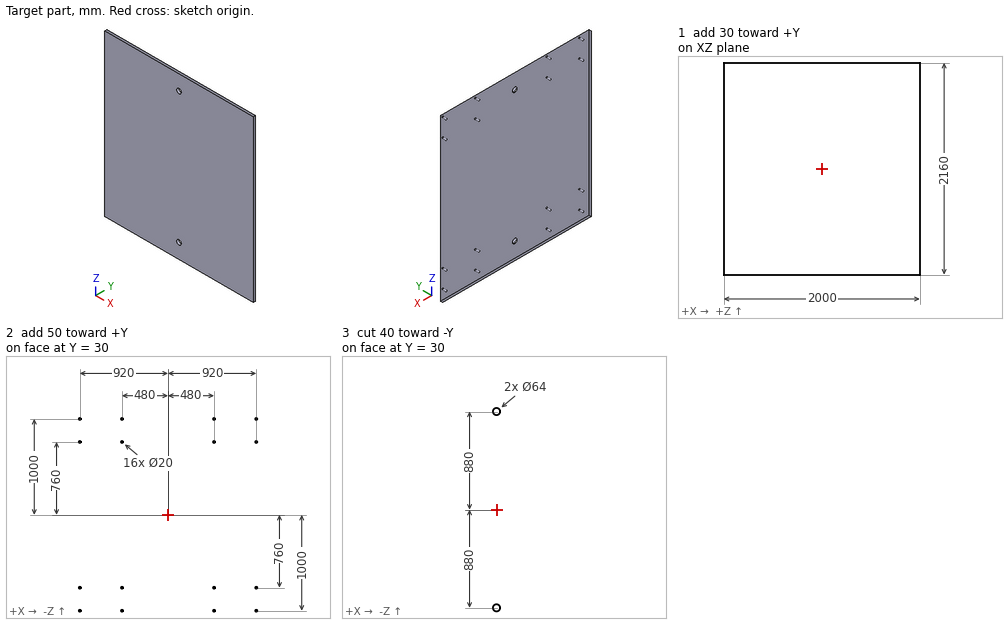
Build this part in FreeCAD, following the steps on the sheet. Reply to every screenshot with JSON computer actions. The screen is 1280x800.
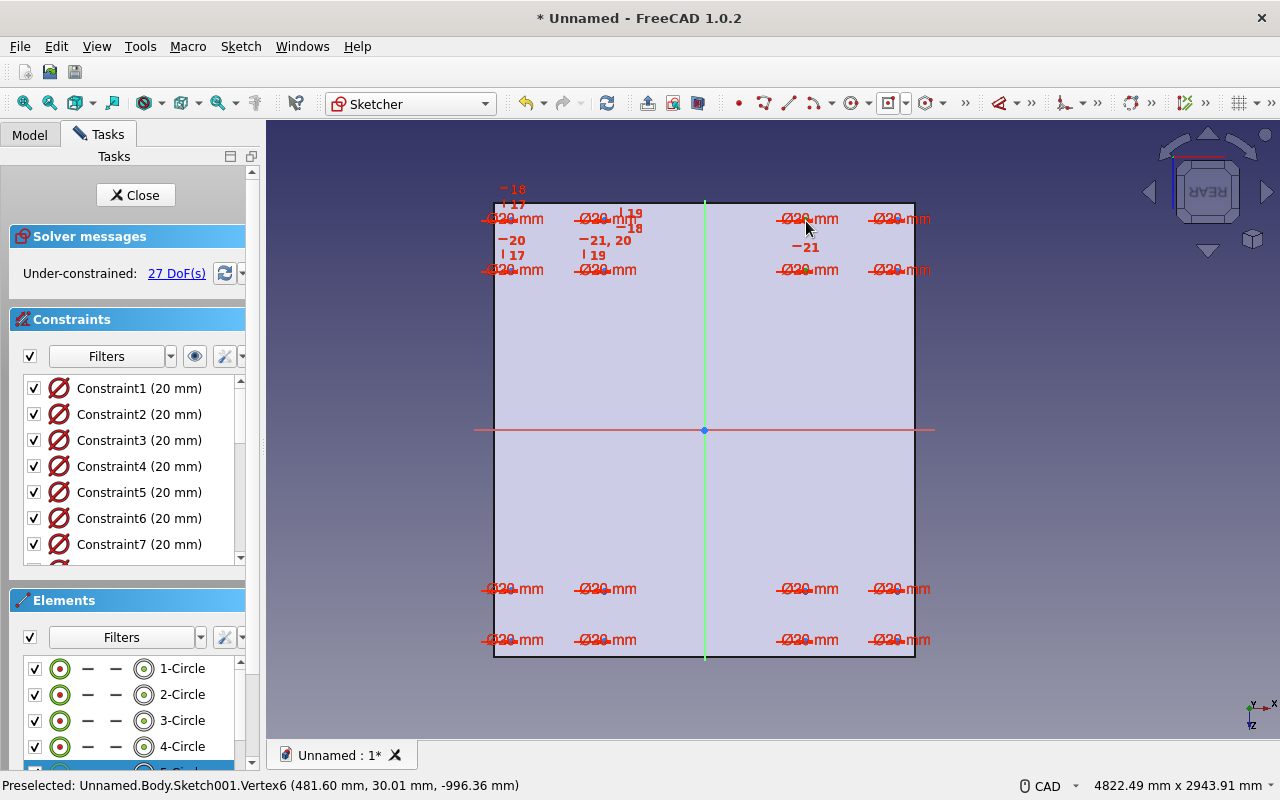
{"action": "key", "text": "v"}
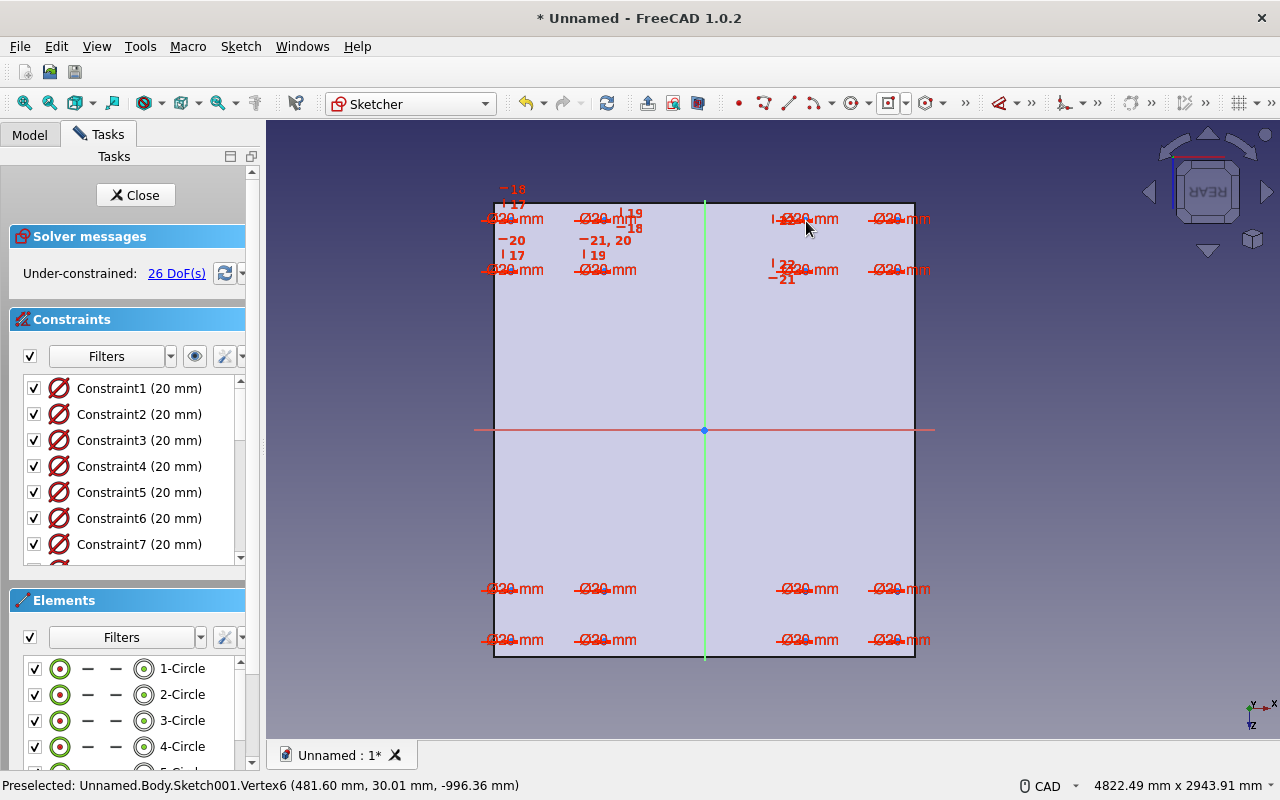
{"action": "left_click", "coordinate": [604, 221]}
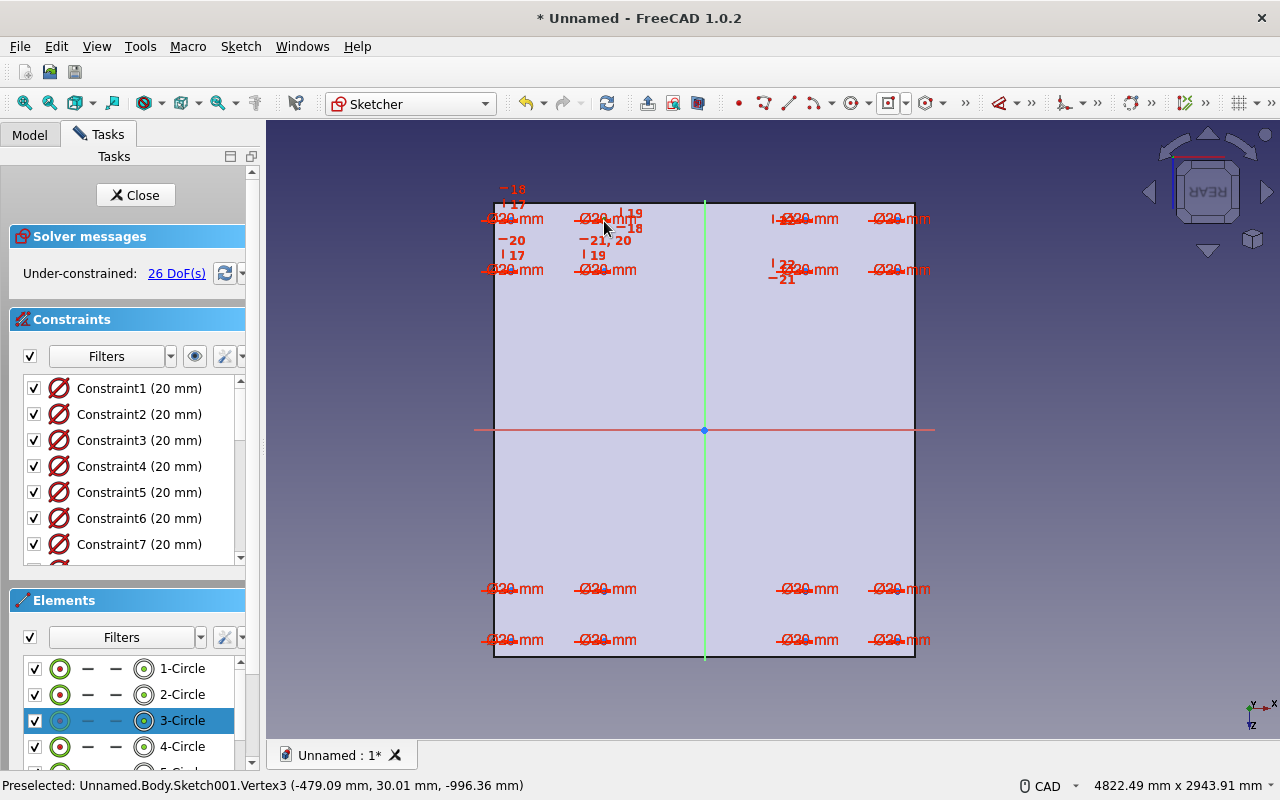
{"action": "left_click", "coordinate": [806, 221]}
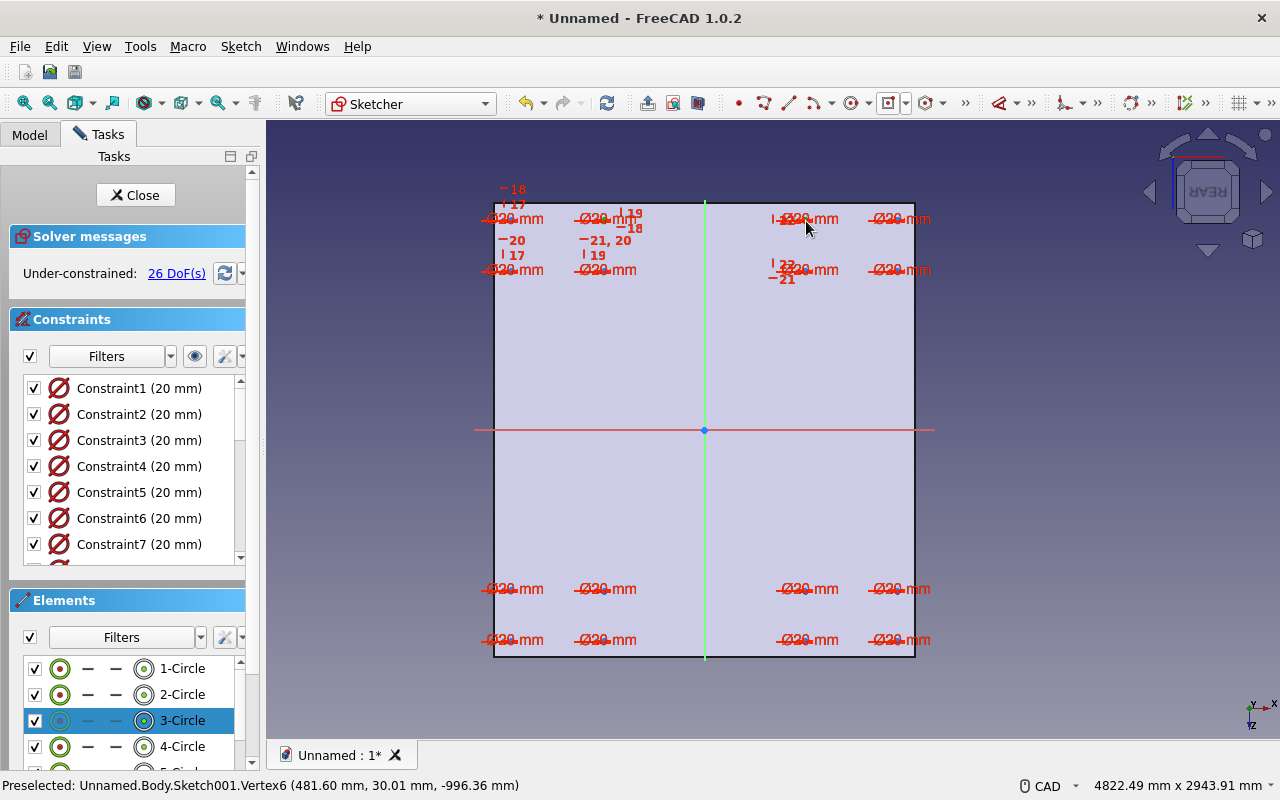
{"action": "key", "text": "h"}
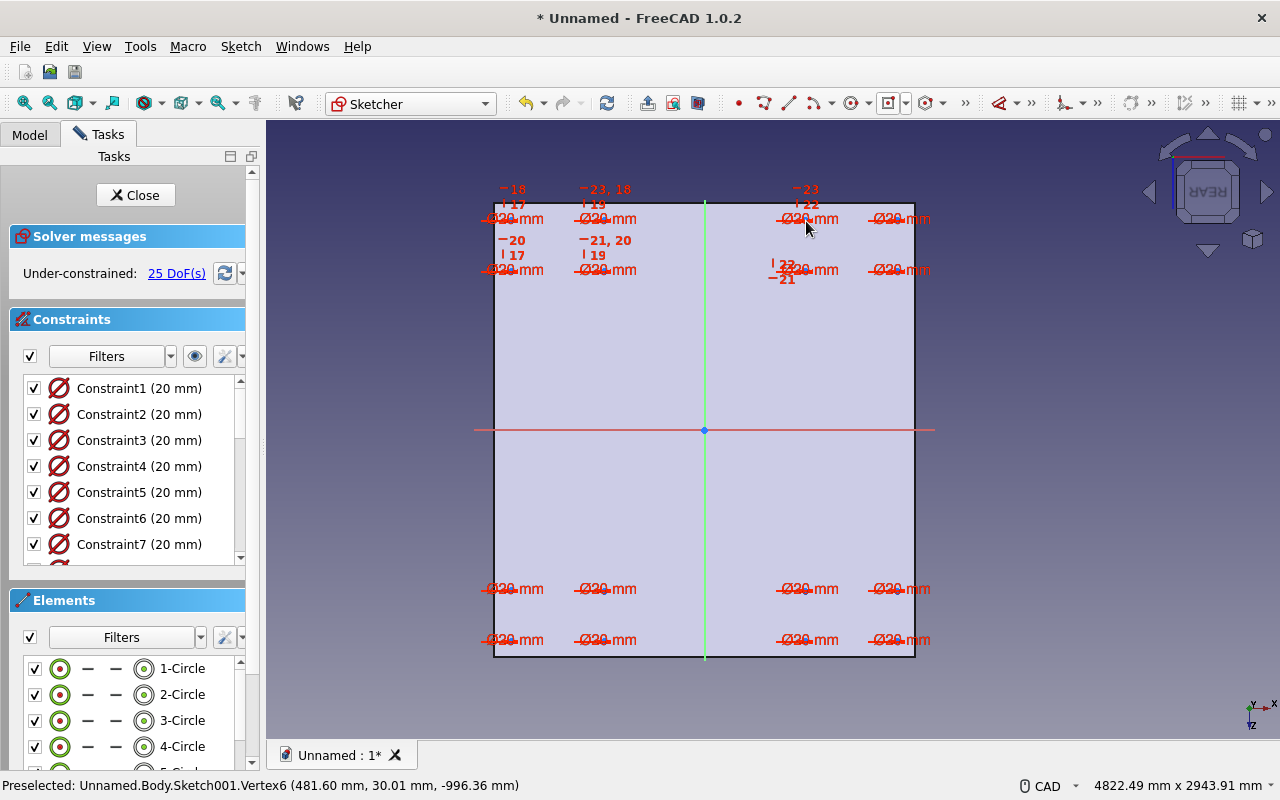
{"action": "left_click", "coordinate": [806, 272]}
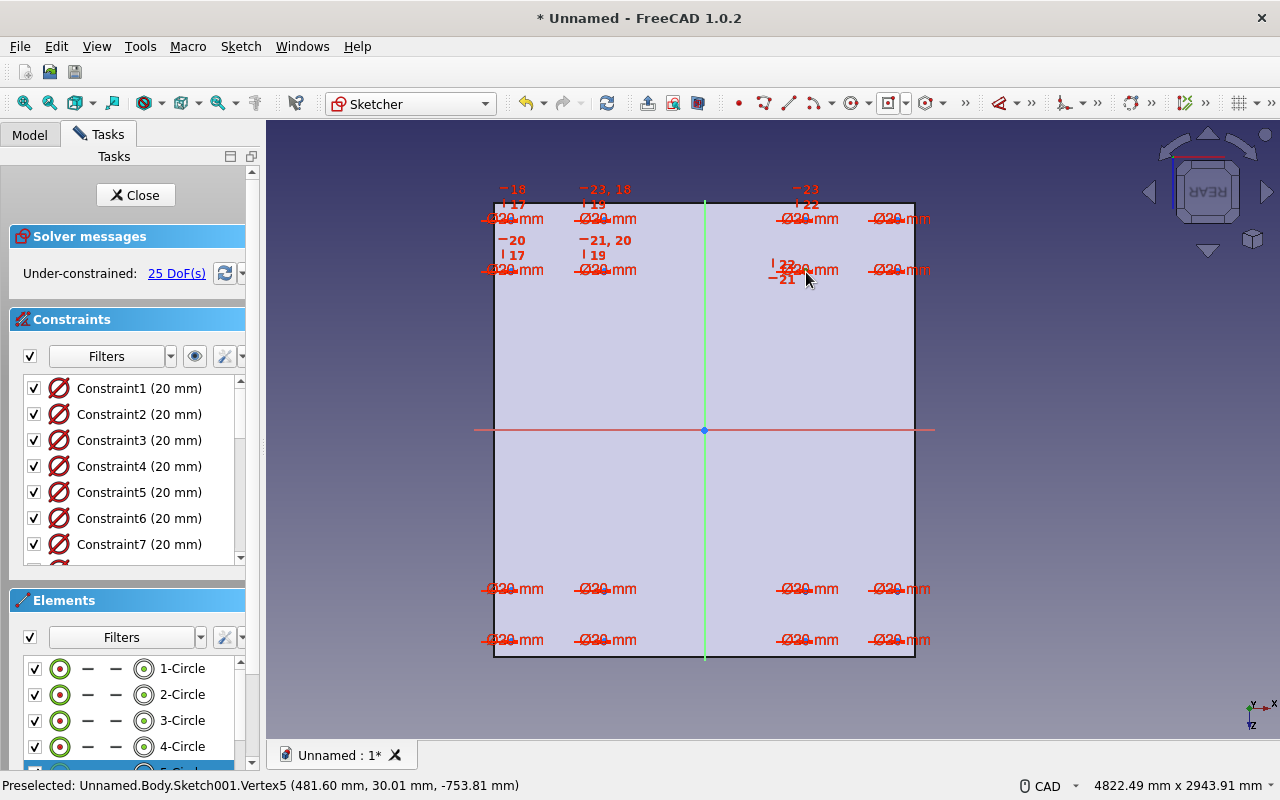
{"action": "left_click", "coordinate": [898, 272]}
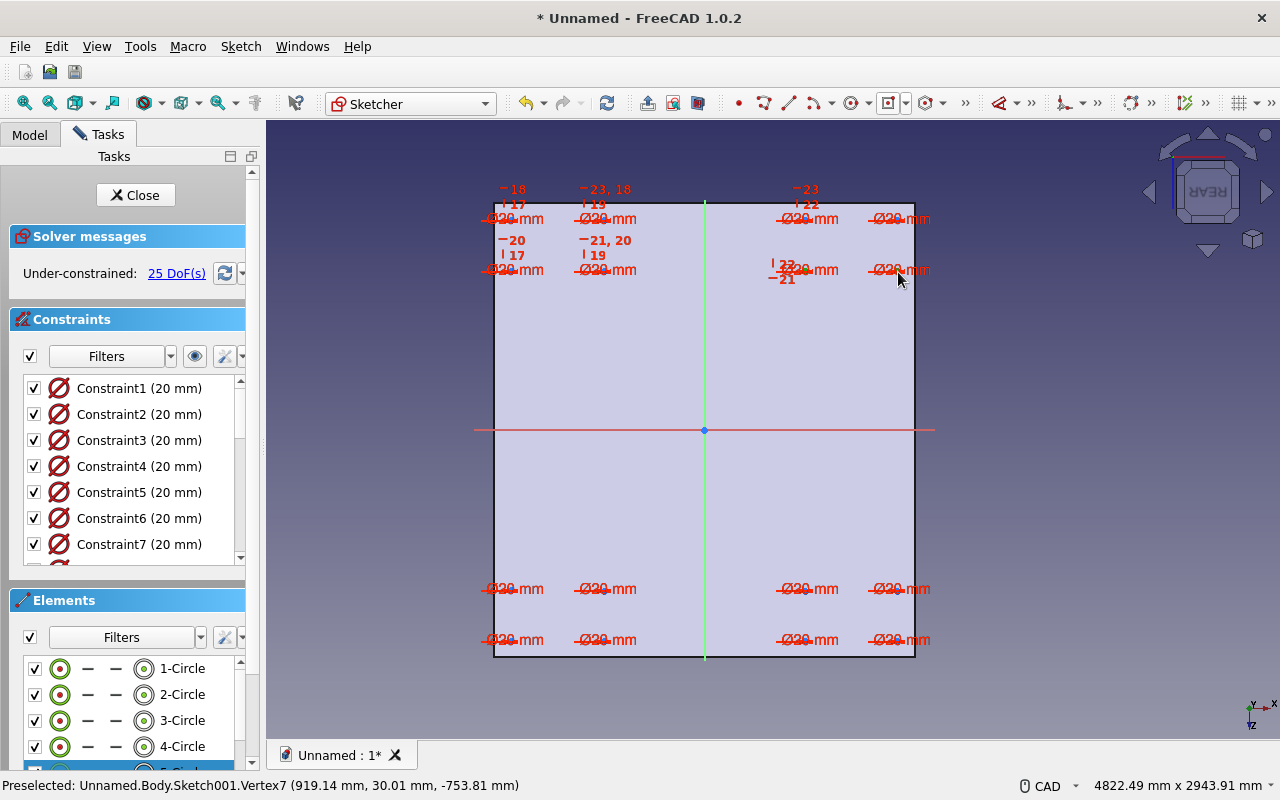
{"action": "key", "text": "h"}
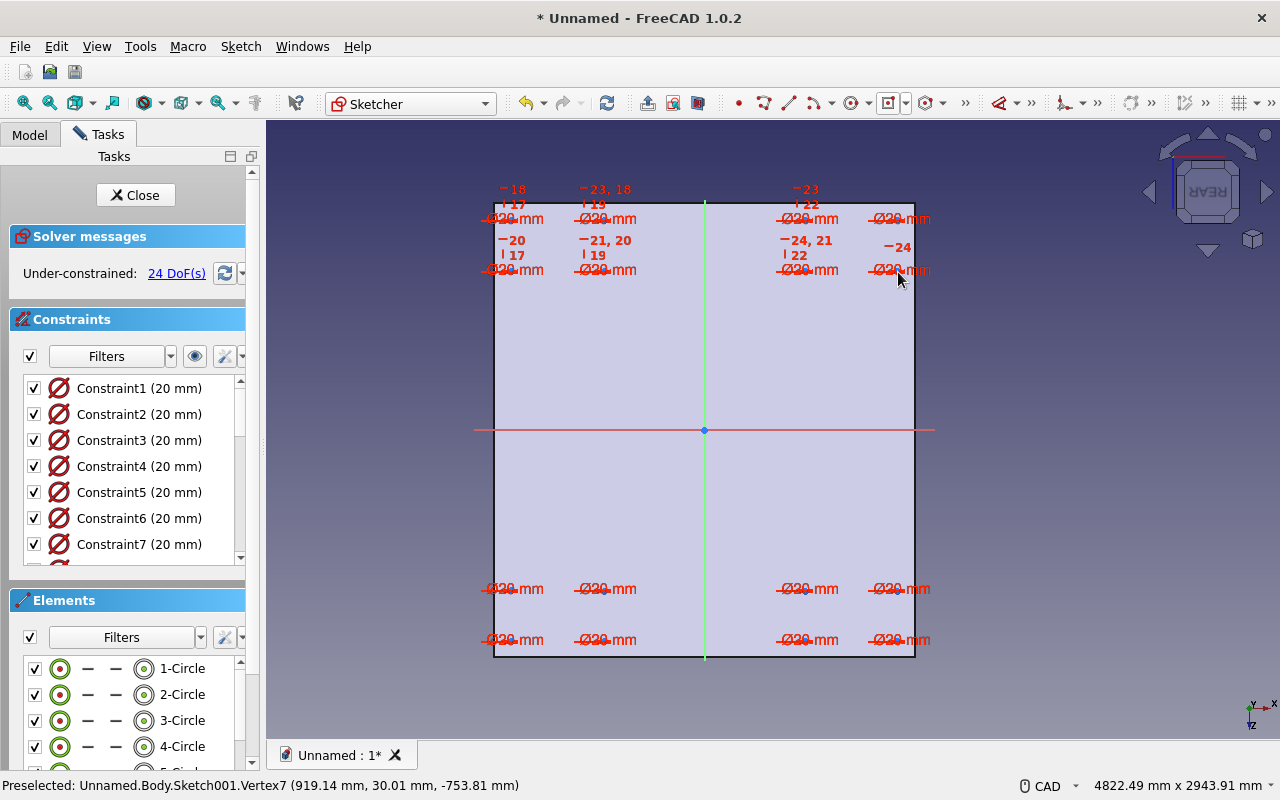
{"action": "left_click", "coordinate": [898, 272]}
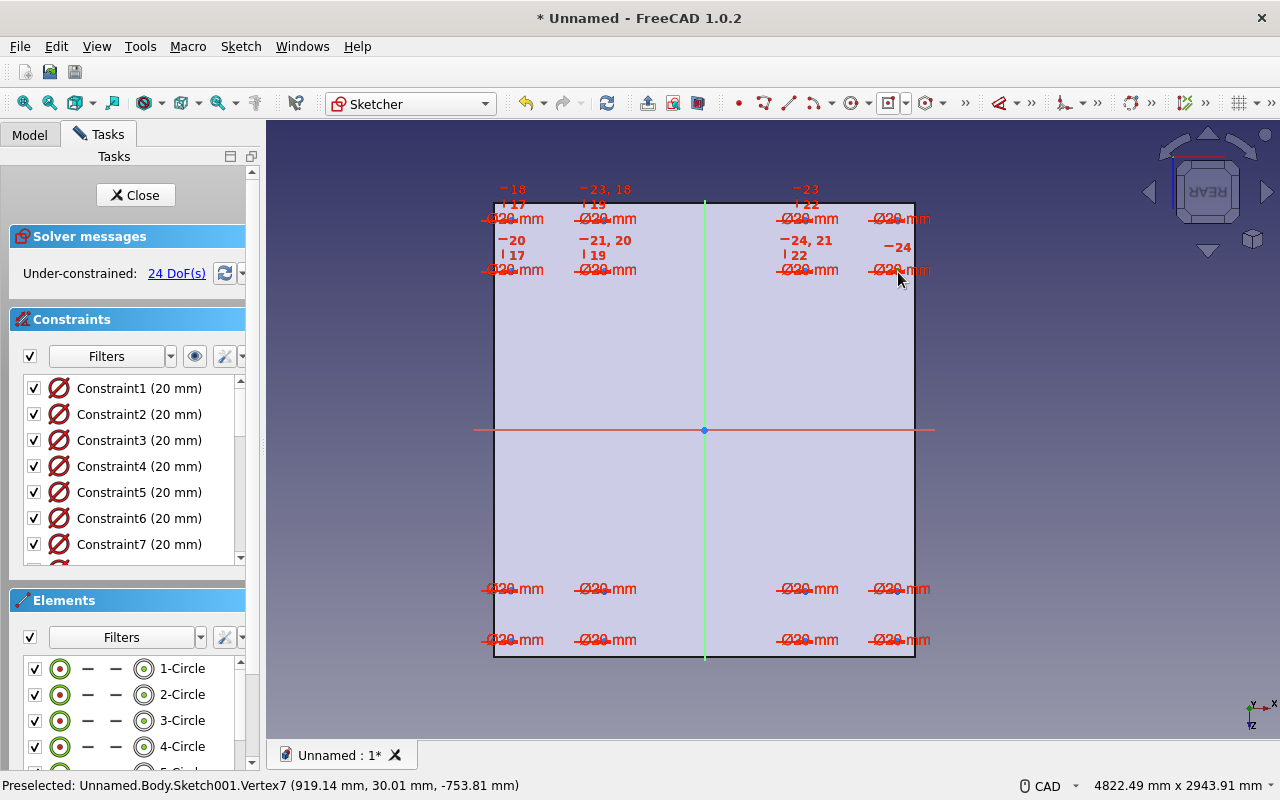
{"action": "left_click", "coordinate": [898, 221]}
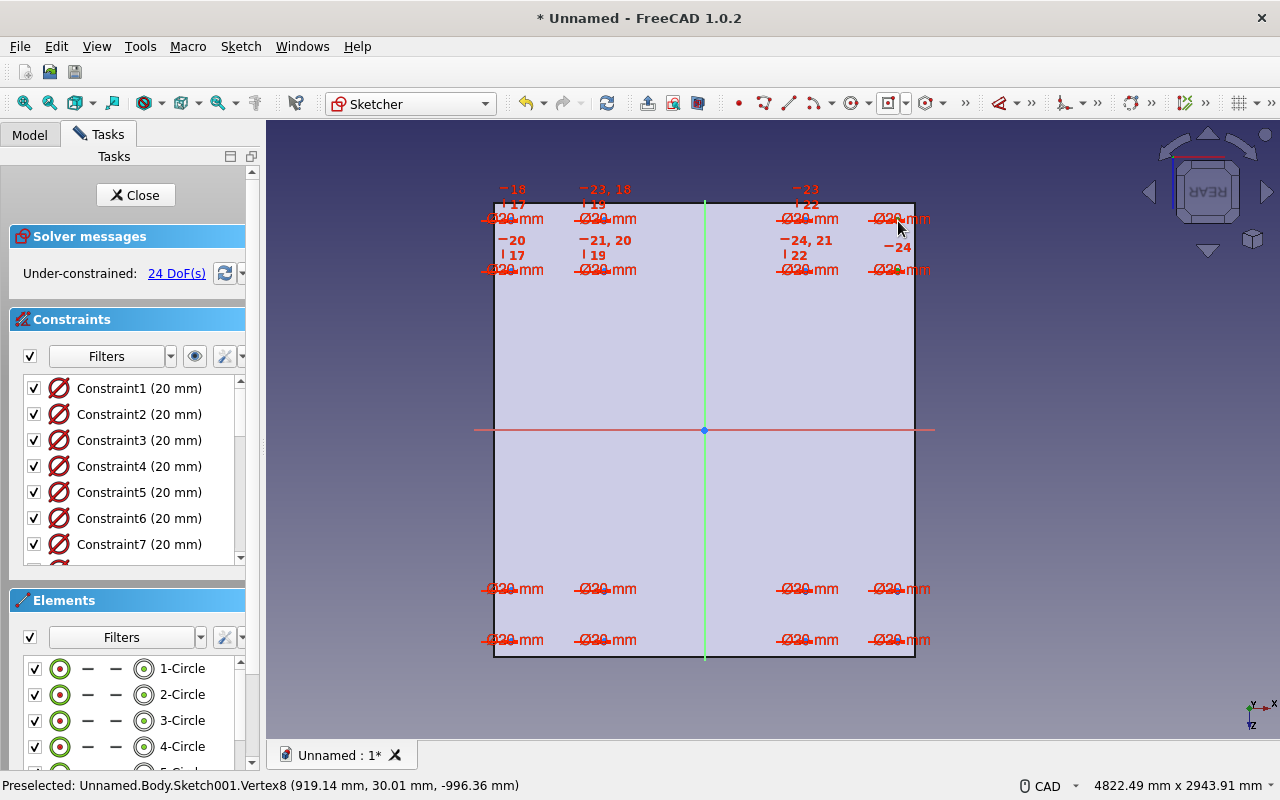
{"action": "key", "text": "v"}